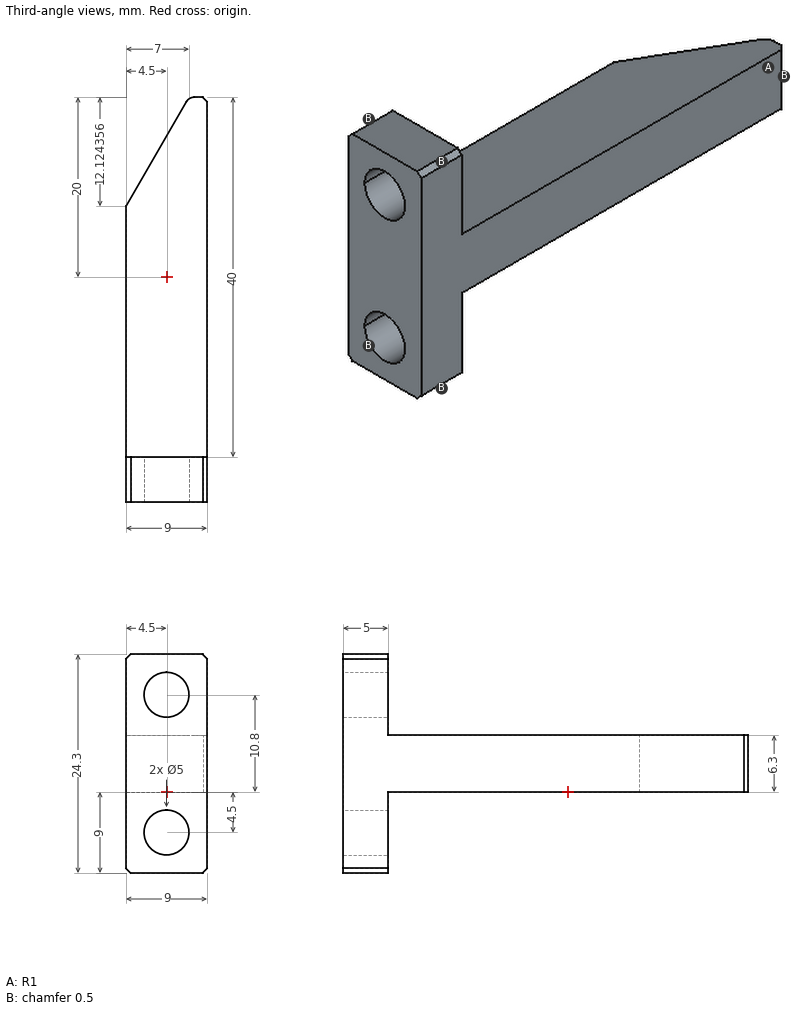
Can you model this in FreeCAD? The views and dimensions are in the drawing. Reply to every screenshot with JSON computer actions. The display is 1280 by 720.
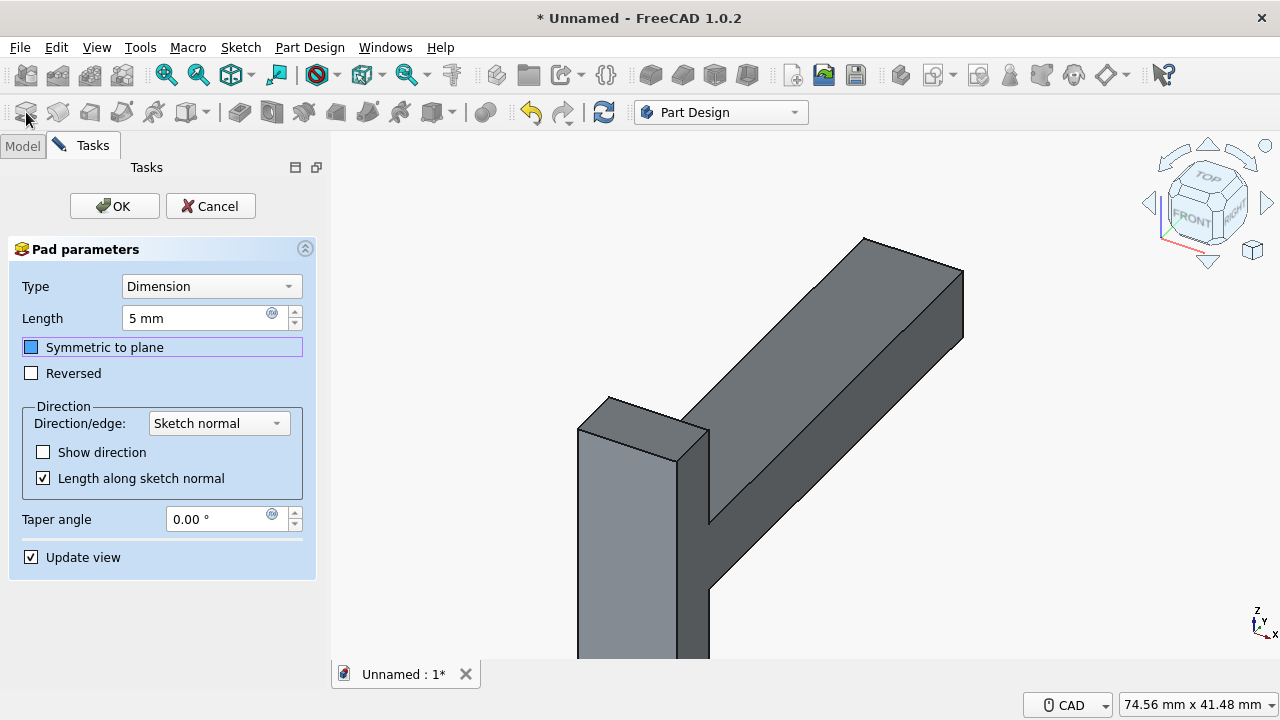
{"action": "left_click", "coordinate": [115, 206]}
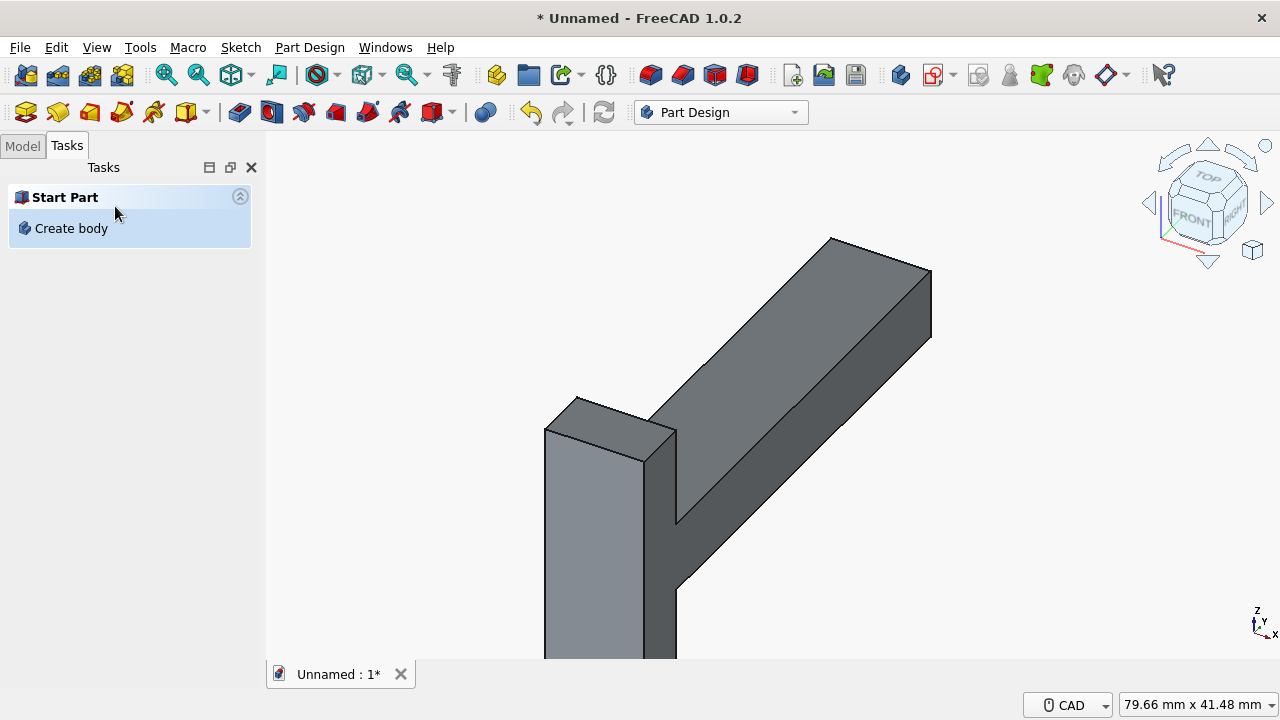
{"action": "left_click", "coordinate": [168, 76]}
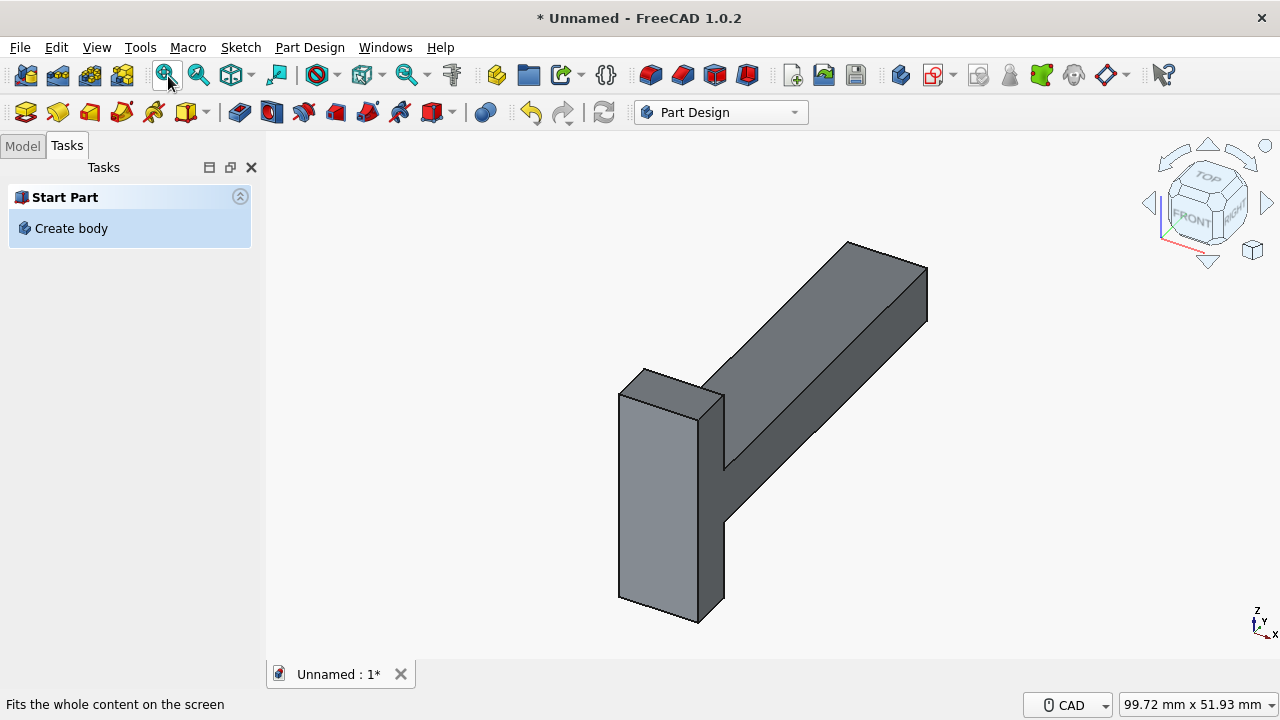
{"action": "key", "text": "5"}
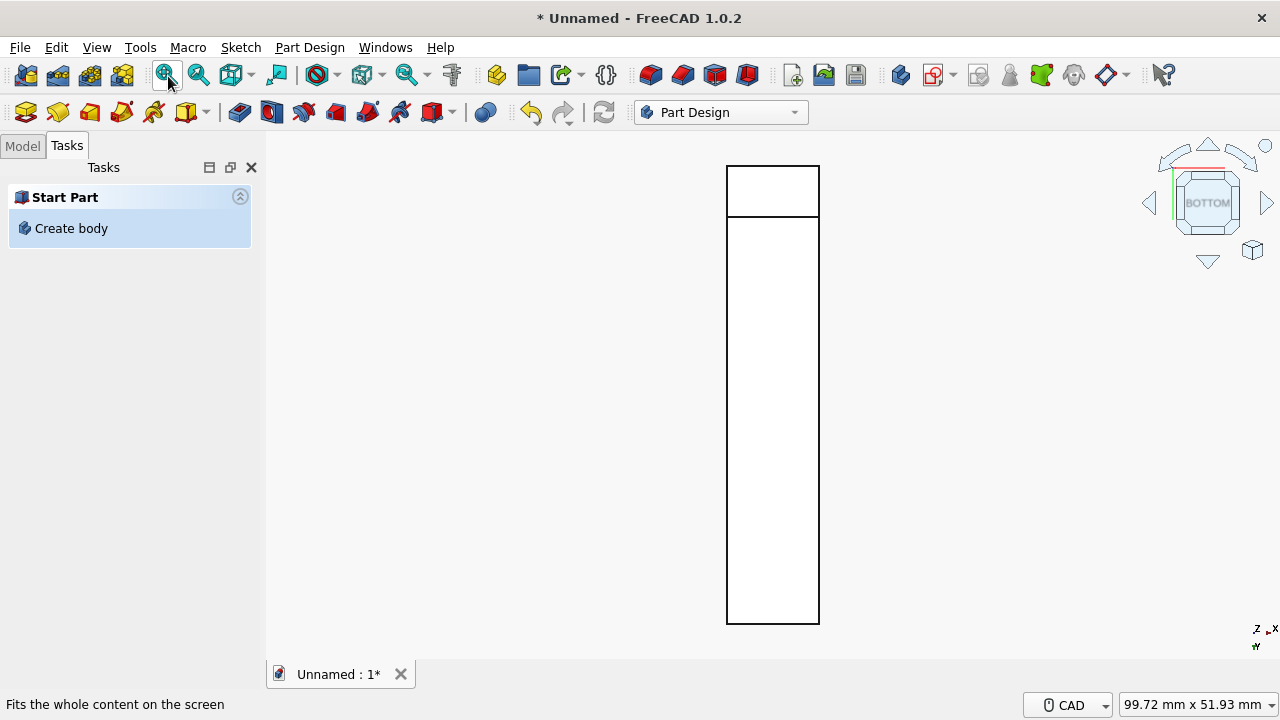
{"action": "left_click", "coordinate": [773, 536]}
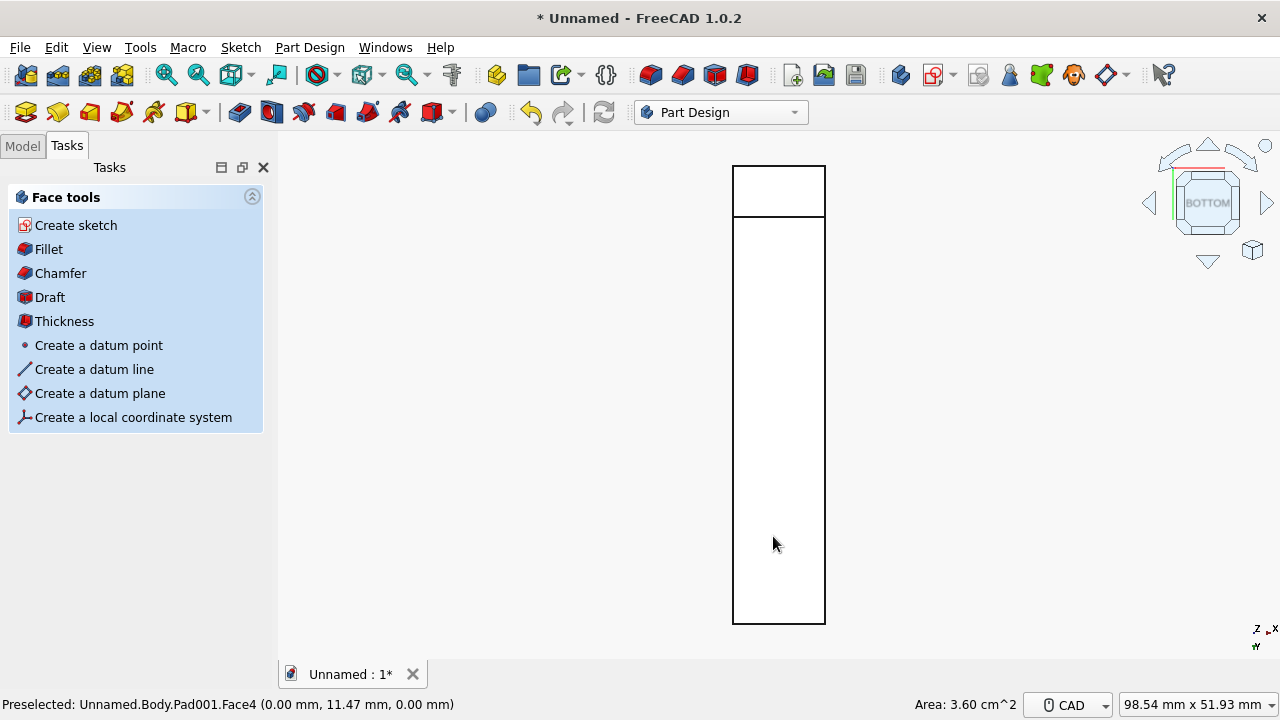
{"action": "left_click", "coordinate": [934, 76]}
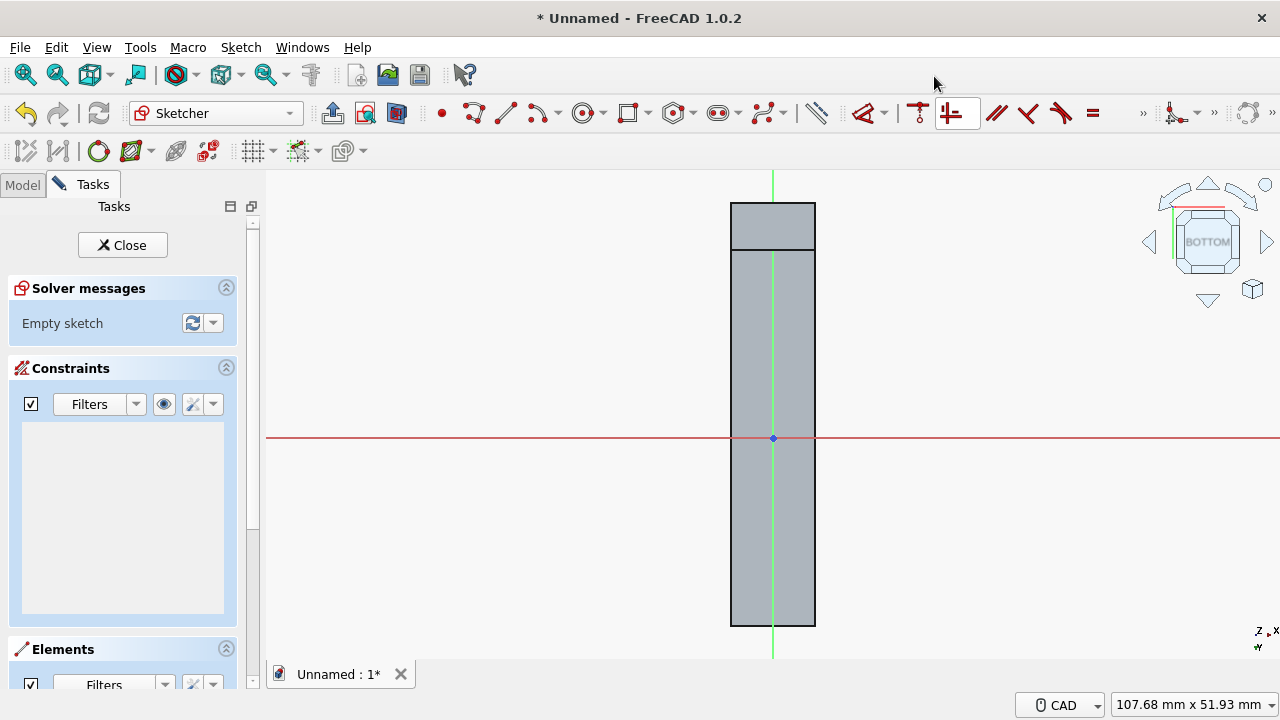
{"action": "scroll", "coordinate": [438, 198], "scroll_direction": "down", "scroll_amount": 1}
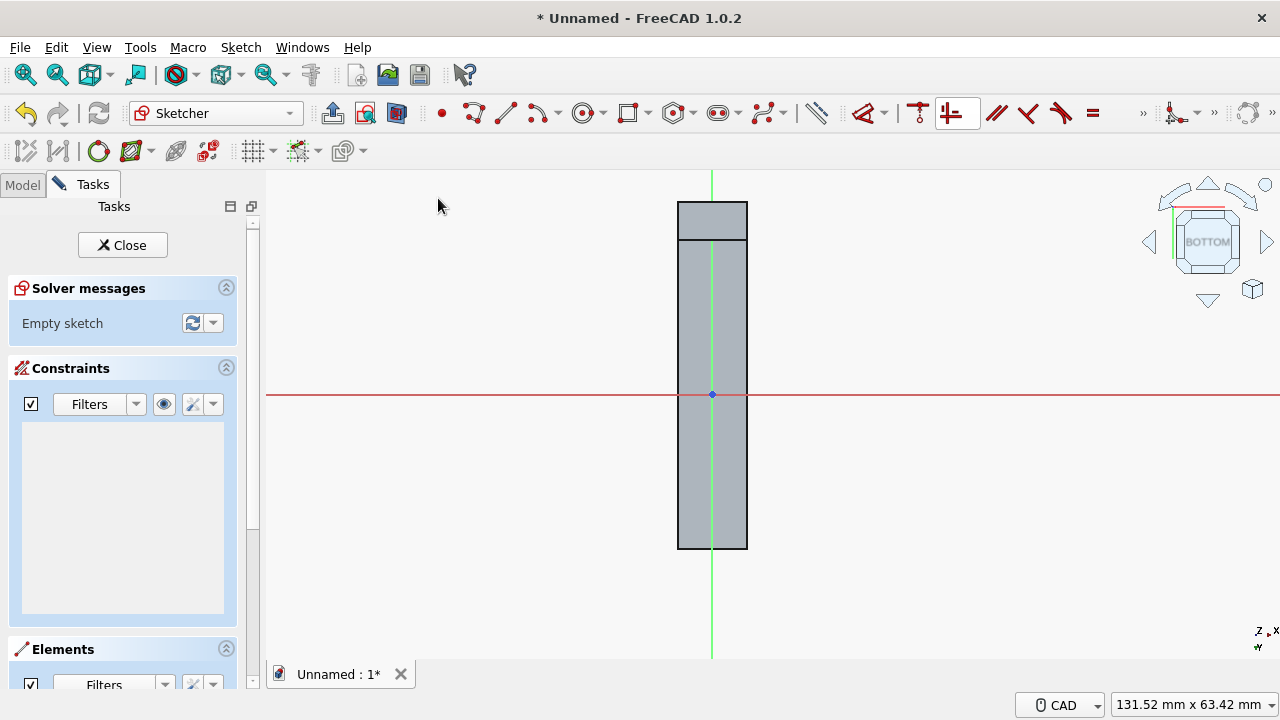
{"action": "scroll", "coordinate": [705, 541], "scroll_direction": "up", "scroll_amount": 3}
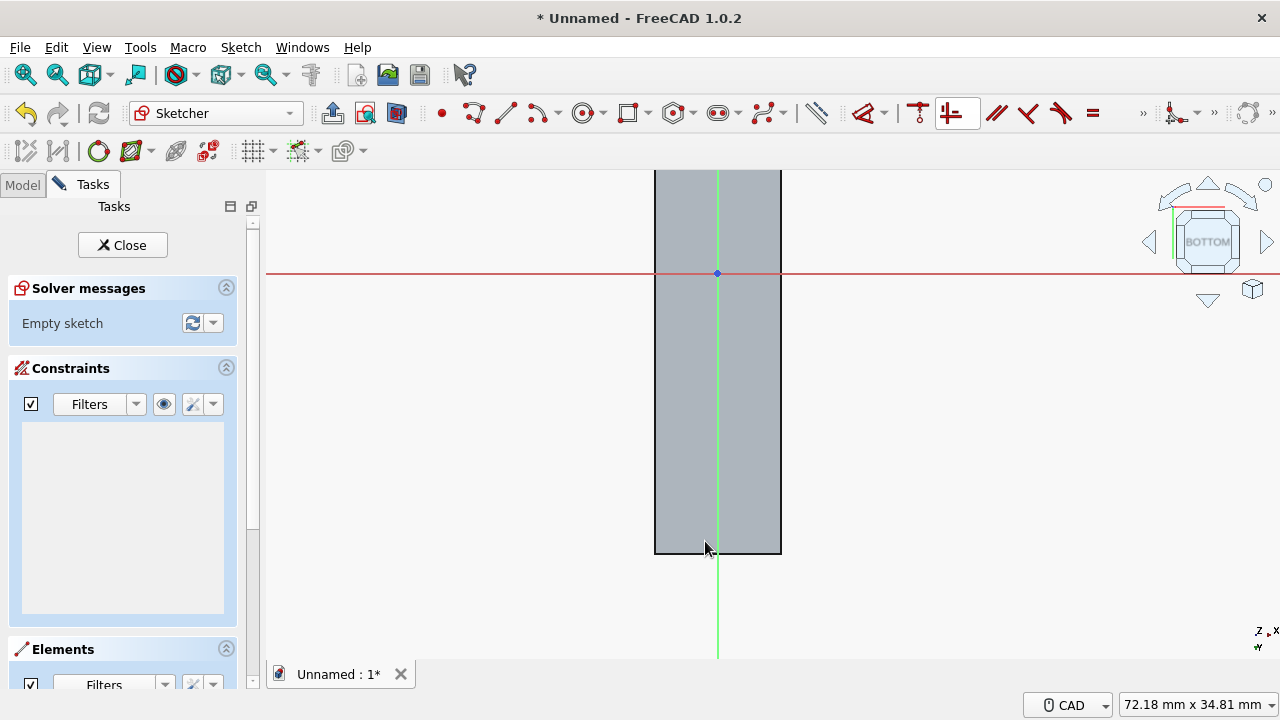
{"action": "key", "text": "g m"}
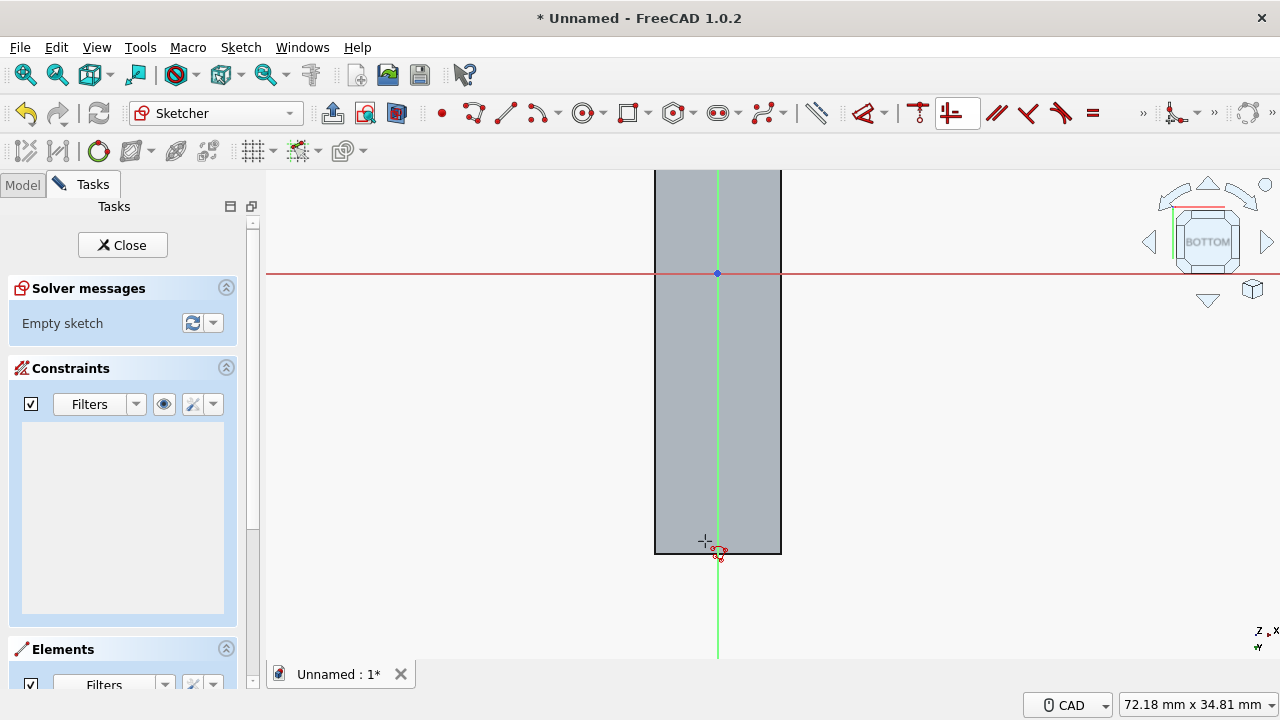
{"action": "left_click", "coordinate": [655, 384]}
{"action": "left_click", "coordinate": [655, 554]}
{"action": "left_click", "coordinate": [753, 554]}
{"action": "left_click", "coordinate": [655, 385]}
{"action": "key", "text": "Escape"}
{"action": "key", "text": "Escape"}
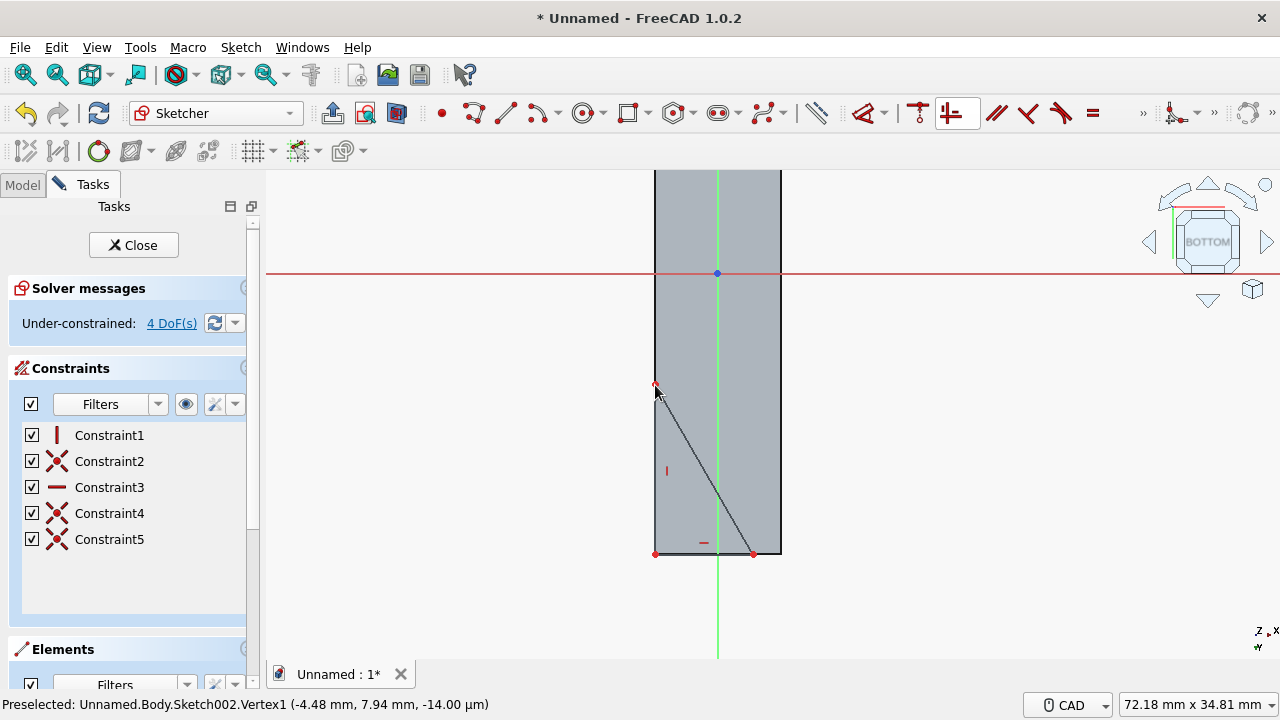
{"action": "key", "text": "d"}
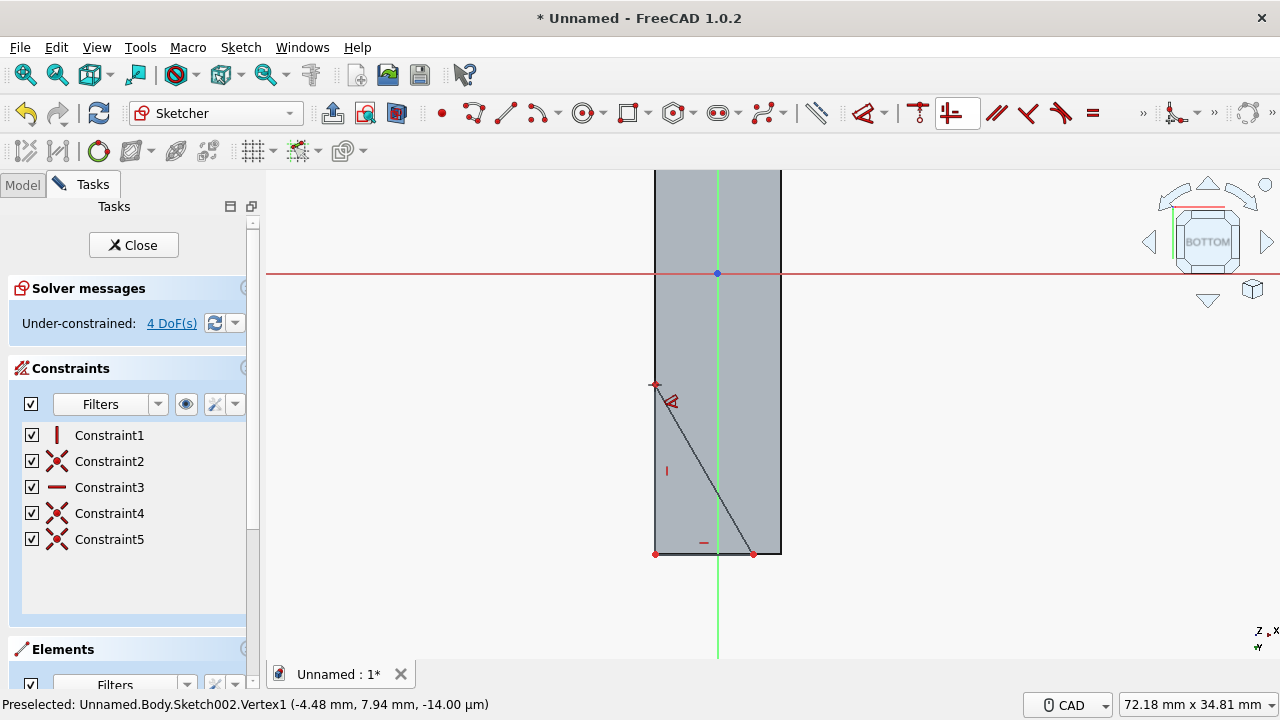
{"action": "left_click", "coordinate": [684, 555]}
{"action": "left_click", "coordinate": [704, 589]}